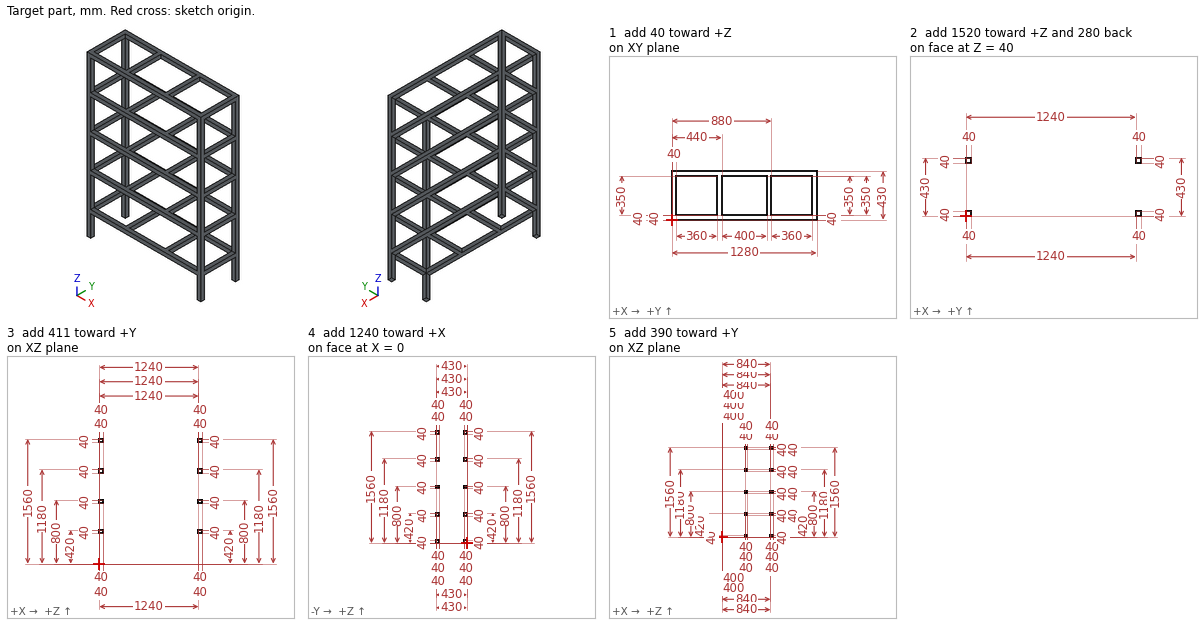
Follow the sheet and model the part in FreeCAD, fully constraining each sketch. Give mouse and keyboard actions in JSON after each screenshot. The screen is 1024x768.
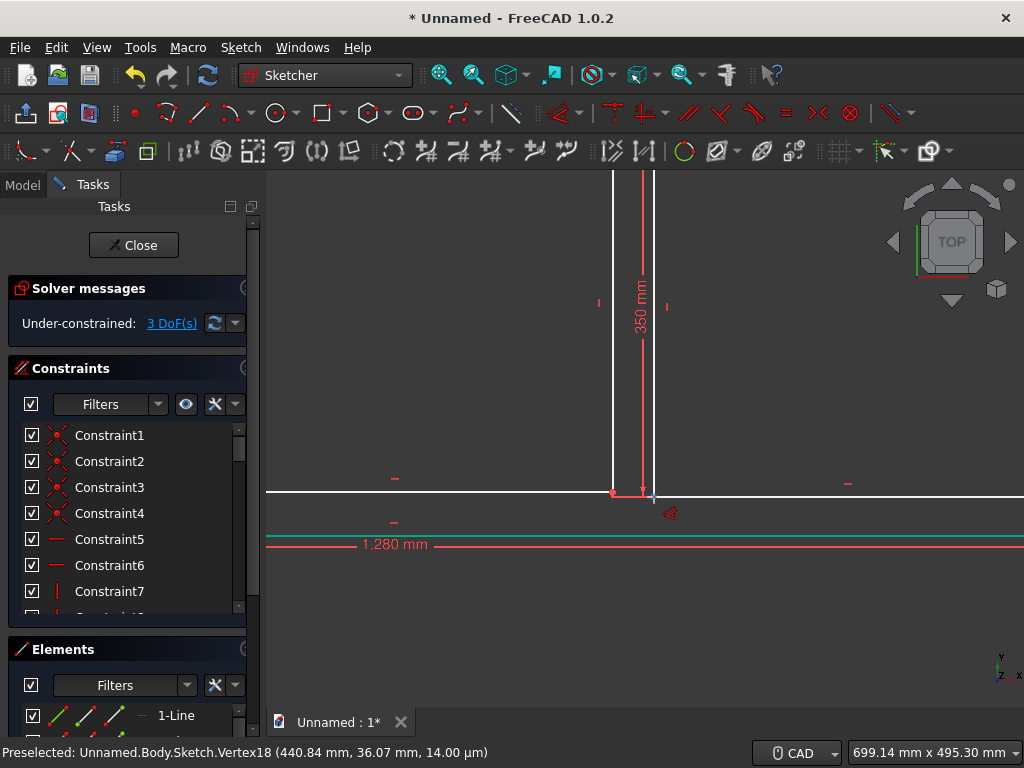
{"action": "left_click", "coordinate": [654, 497]}
{"action": "left_click", "coordinate": [688, 516]}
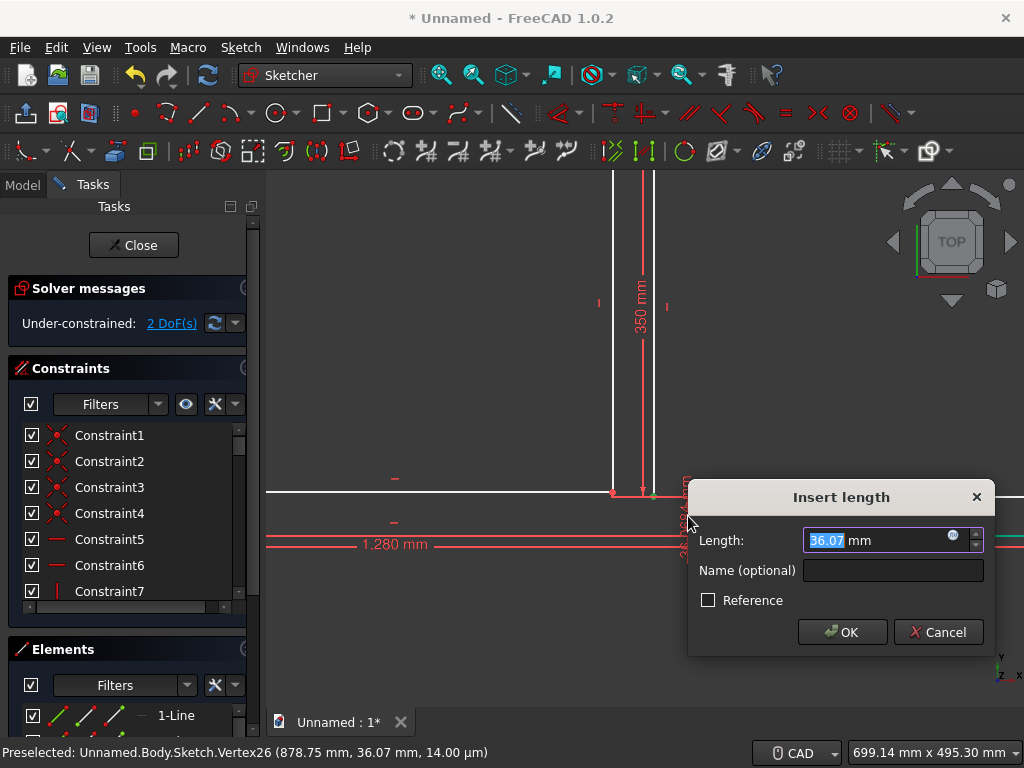
{"action": "type", "text": "40"}
{"action": "key", "text": "Return"}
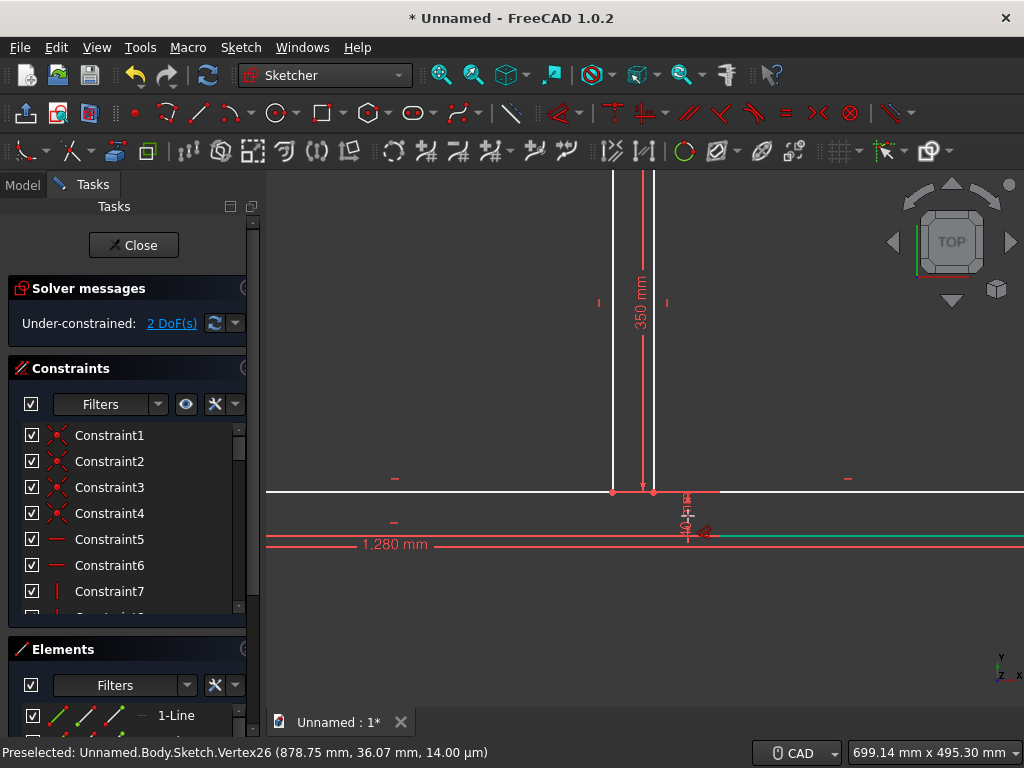
{"action": "scroll", "coordinate": [655, 497], "scroll_direction": "down", "scroll_amount": 6}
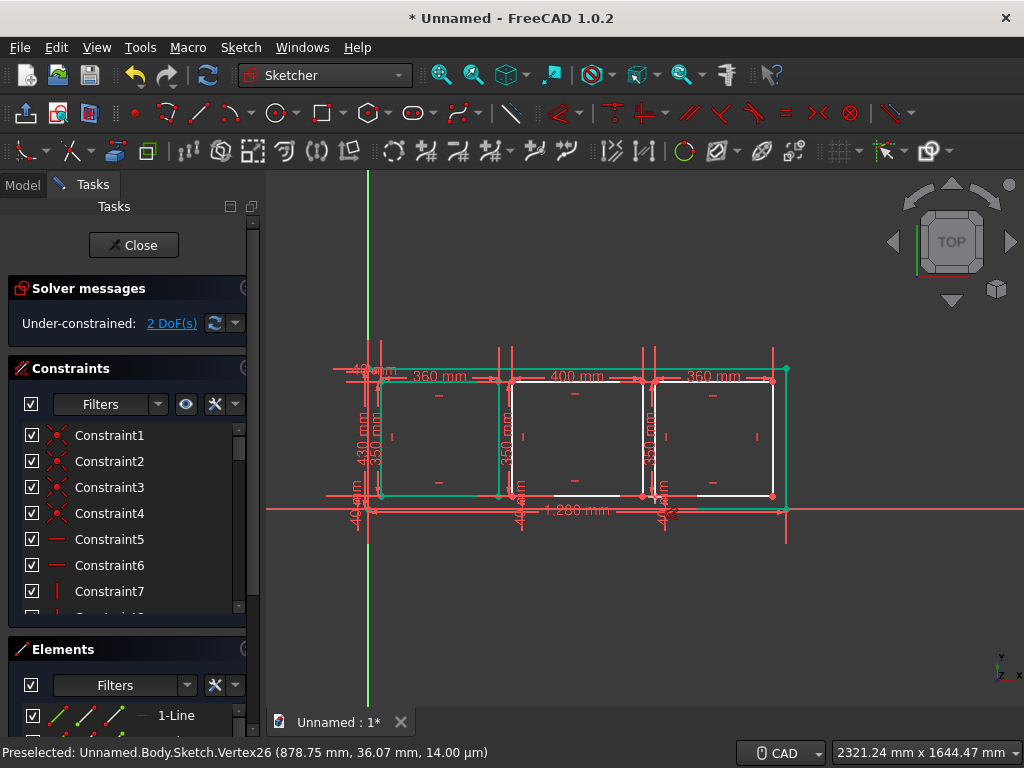
{"action": "left_click", "coordinate": [512, 382]}
{"action": "left_click", "coordinate": [440, 543]}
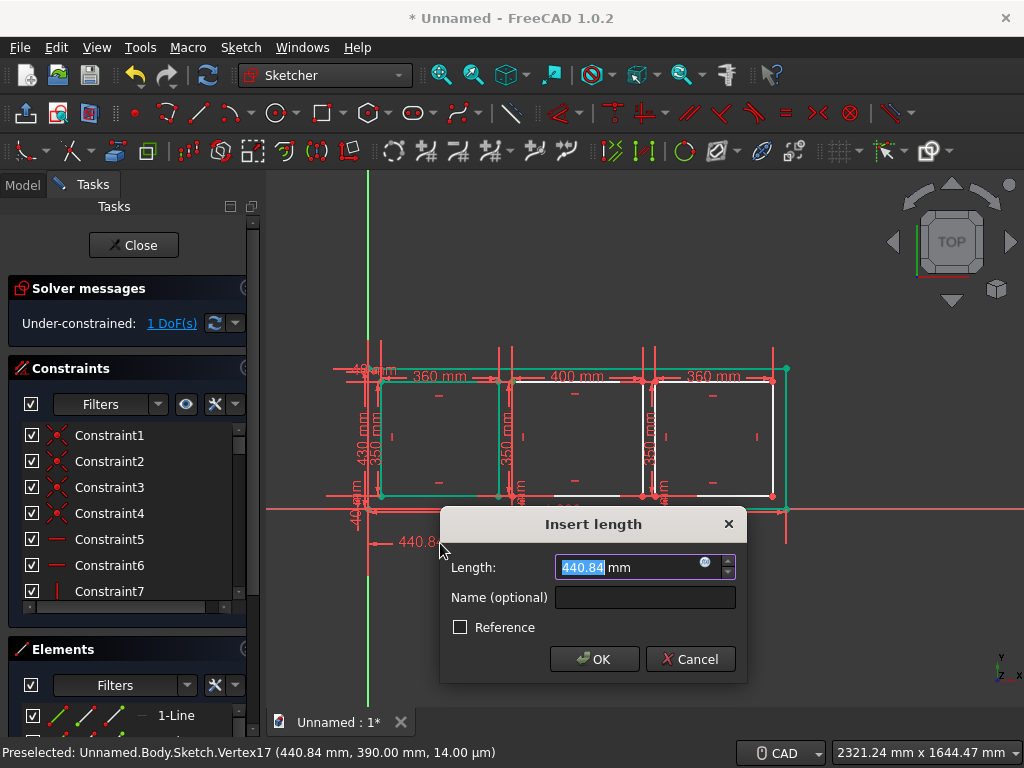
{"action": "type", "text": "440"}
{"action": "key", "text": "Return"}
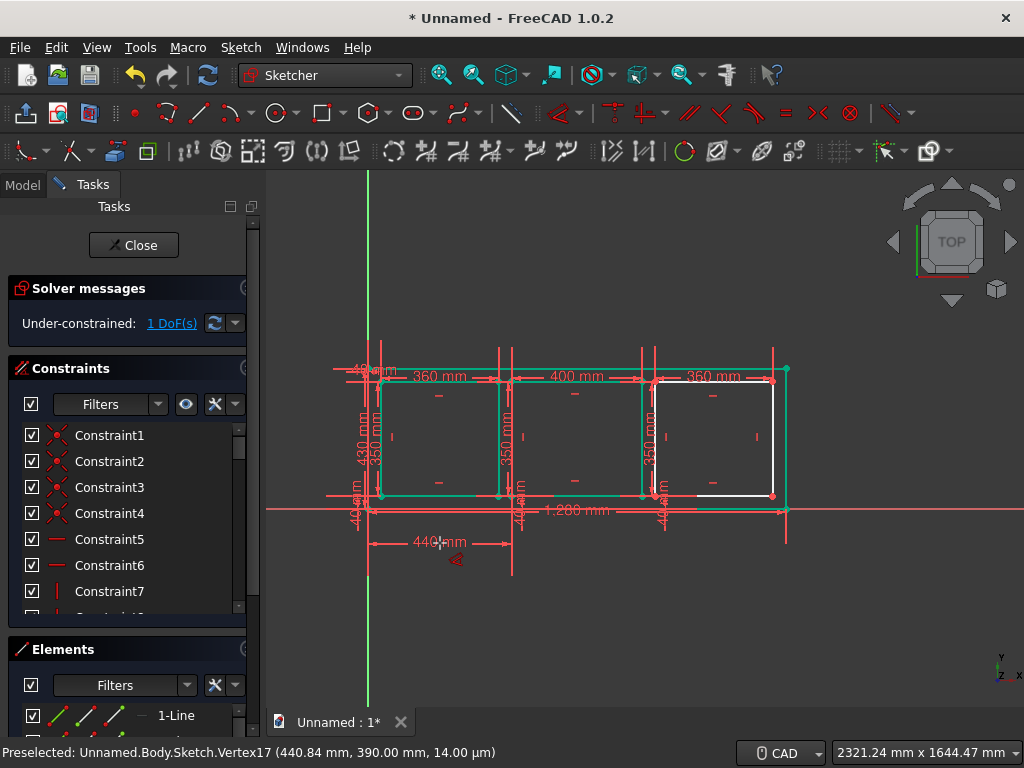
{"action": "left_click", "coordinate": [655, 382]}
{"action": "left_click", "coordinate": [512, 543]}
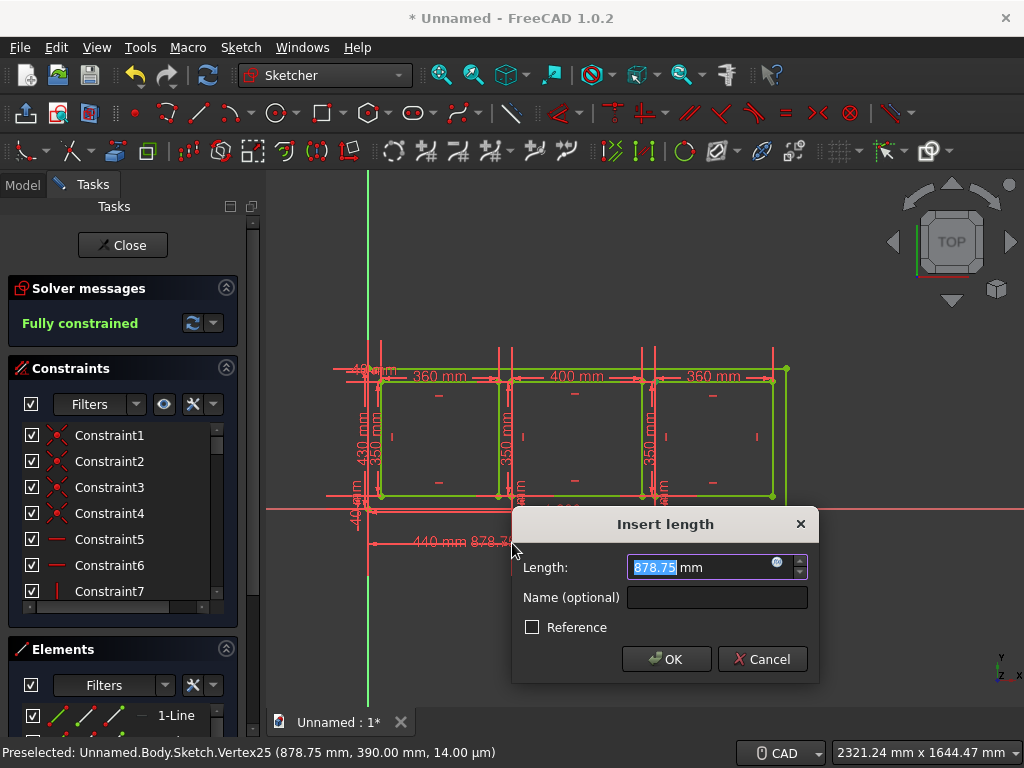
{"action": "type", "text": "880"}
{"action": "key", "text": "Return"}
{"action": "key", "text": "Escape"}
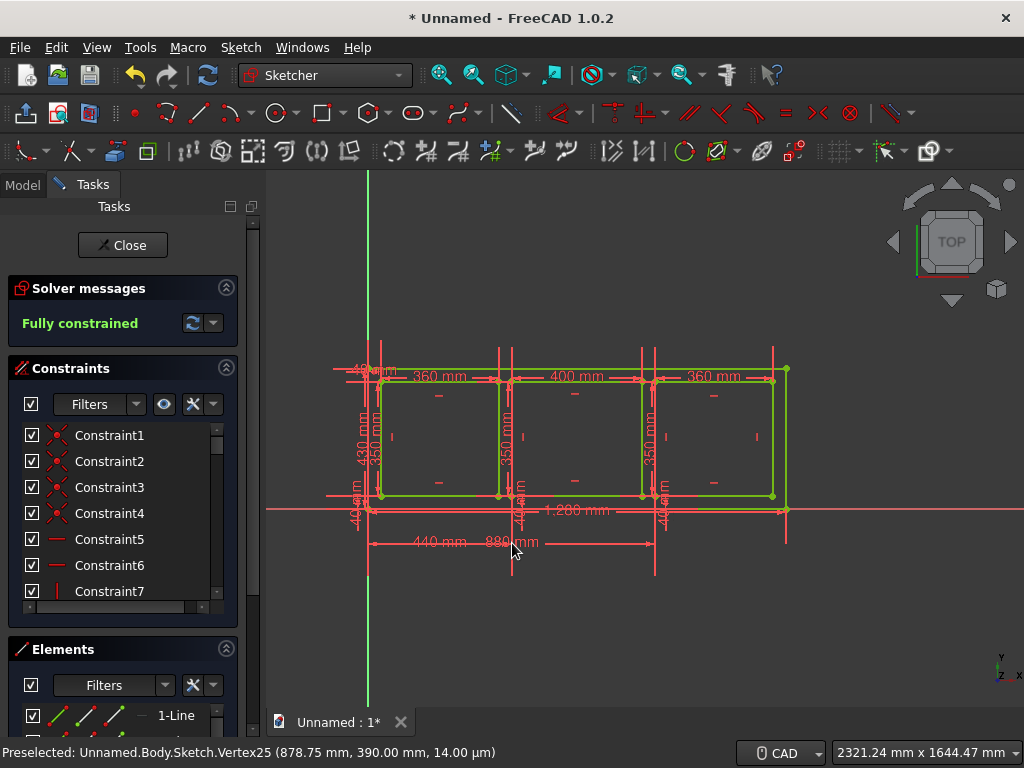
{"action": "left_click", "coordinate": [123, 245]}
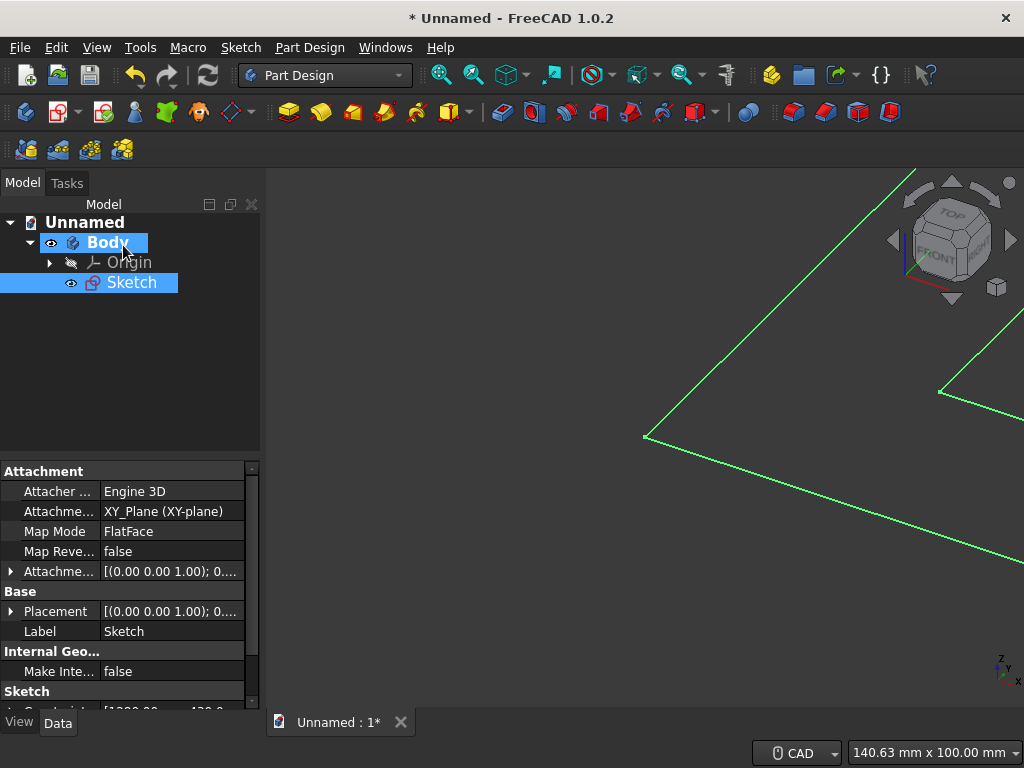
{"action": "left_click", "coordinate": [290, 112]}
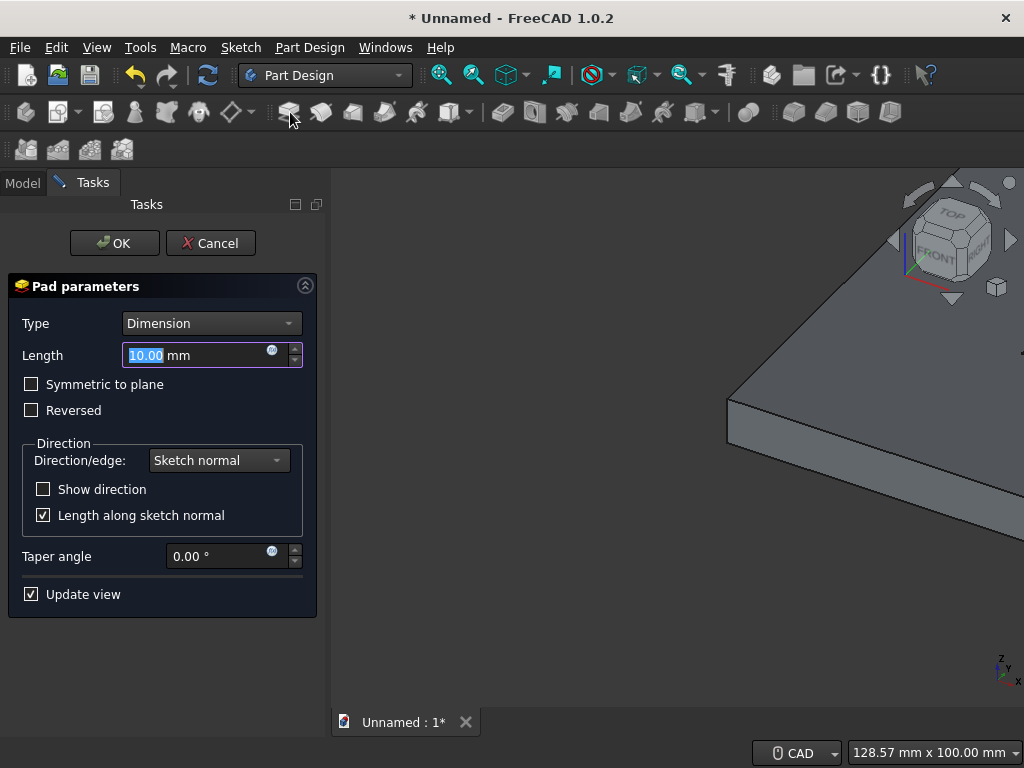
{"action": "type", "text": "40"}
{"action": "key", "text": "Tab"}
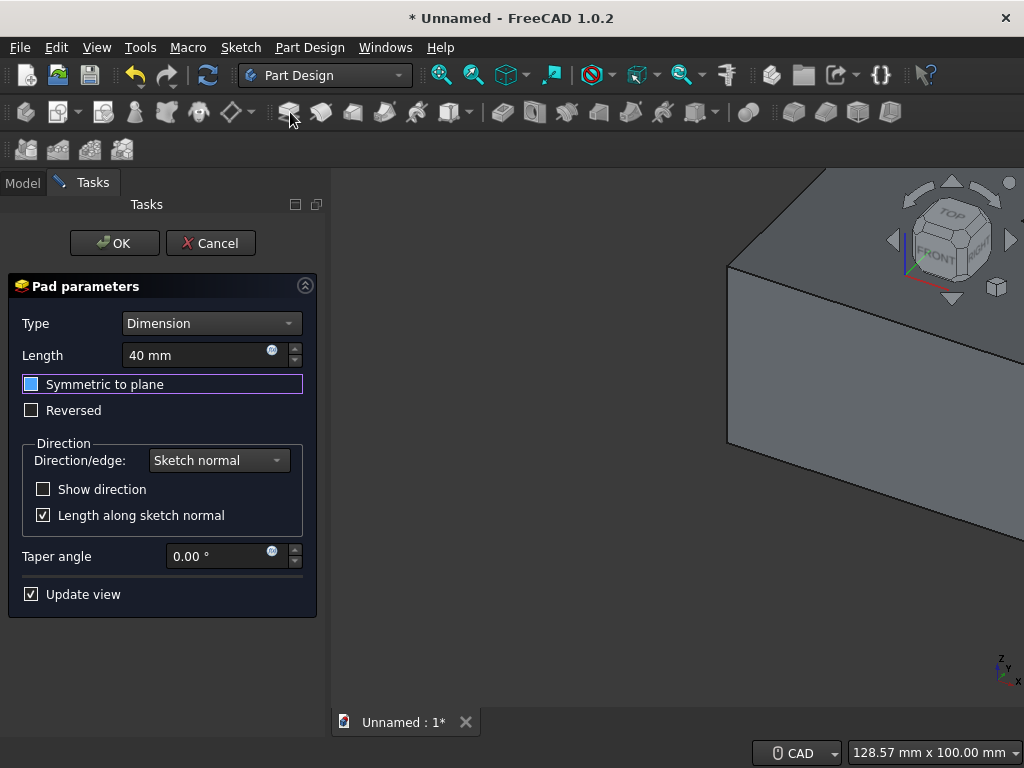
{"action": "left_click", "coordinate": [115, 243]}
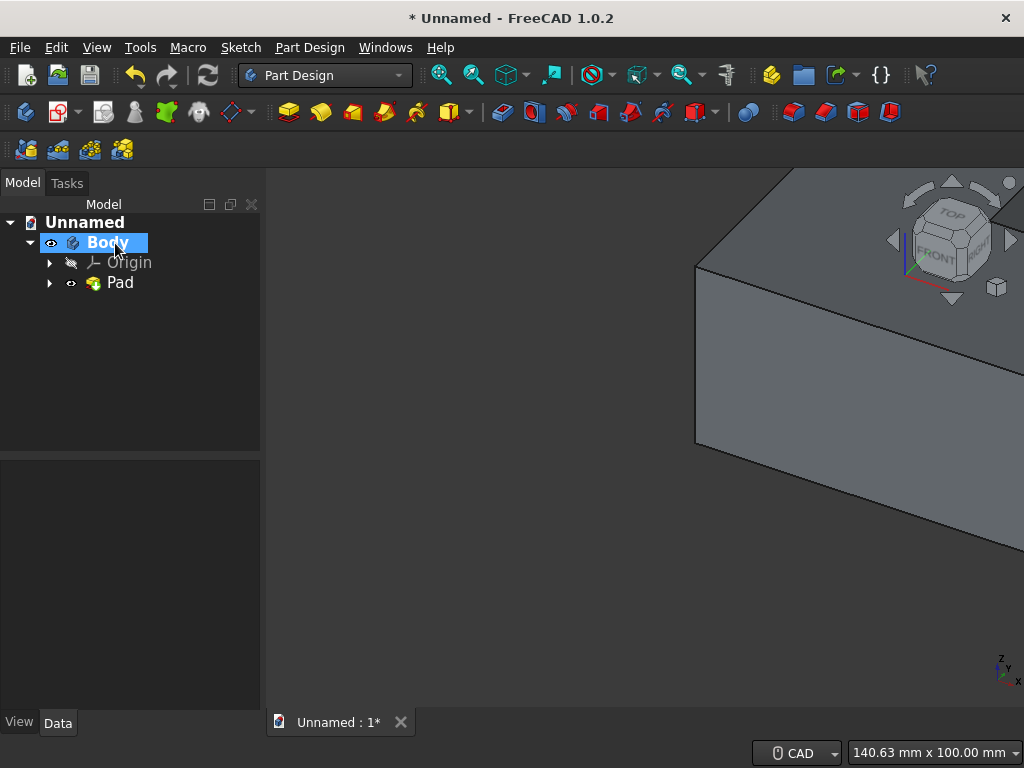
{"action": "left_click", "coordinate": [442, 76]}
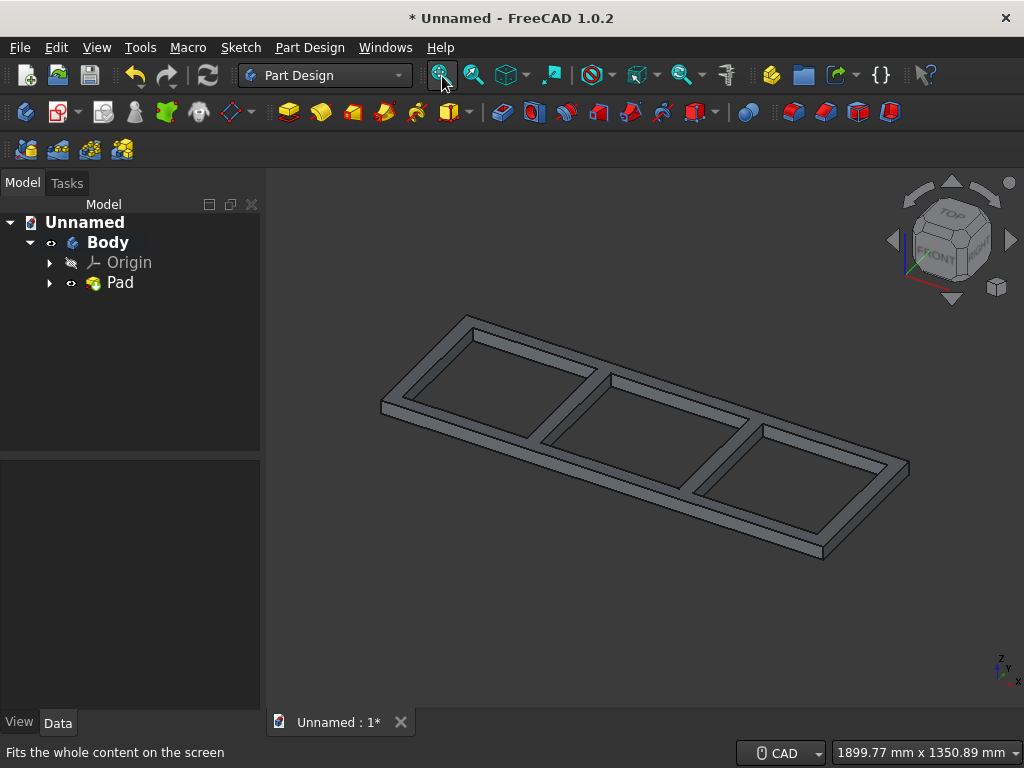
{"action": "key", "text": "0"}